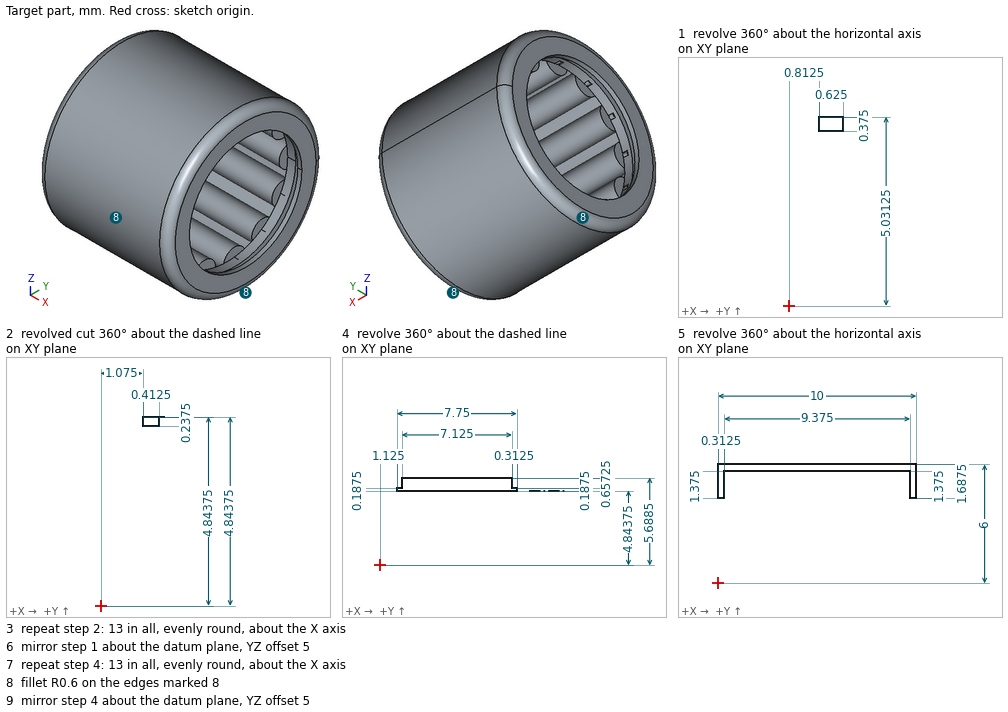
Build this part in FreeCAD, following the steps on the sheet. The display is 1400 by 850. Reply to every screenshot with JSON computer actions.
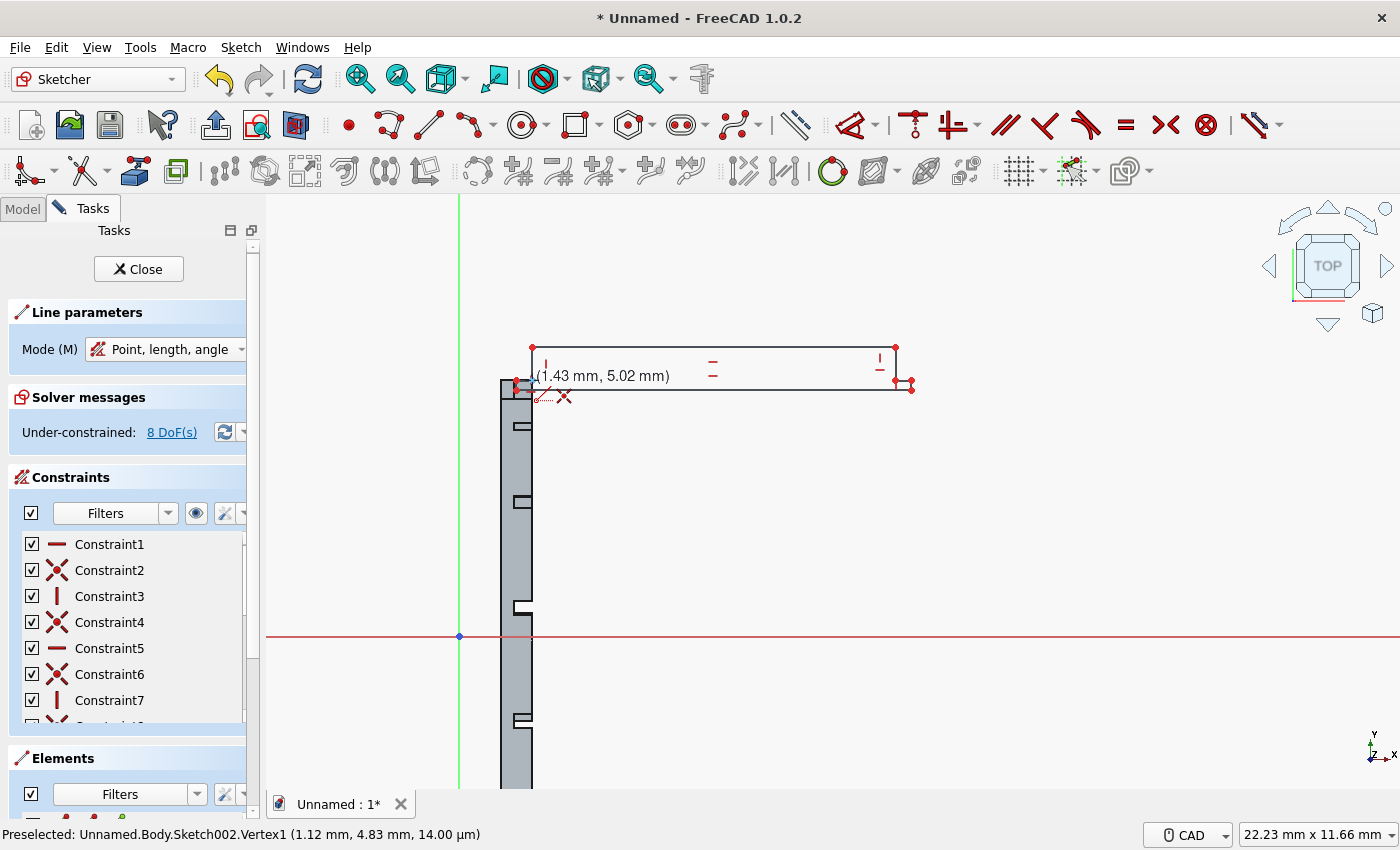
{"action": "left_click", "coordinate": [951, 390]}
{"action": "left_click", "coordinate": [1070, 390]}
{"action": "key", "text": "Escape"}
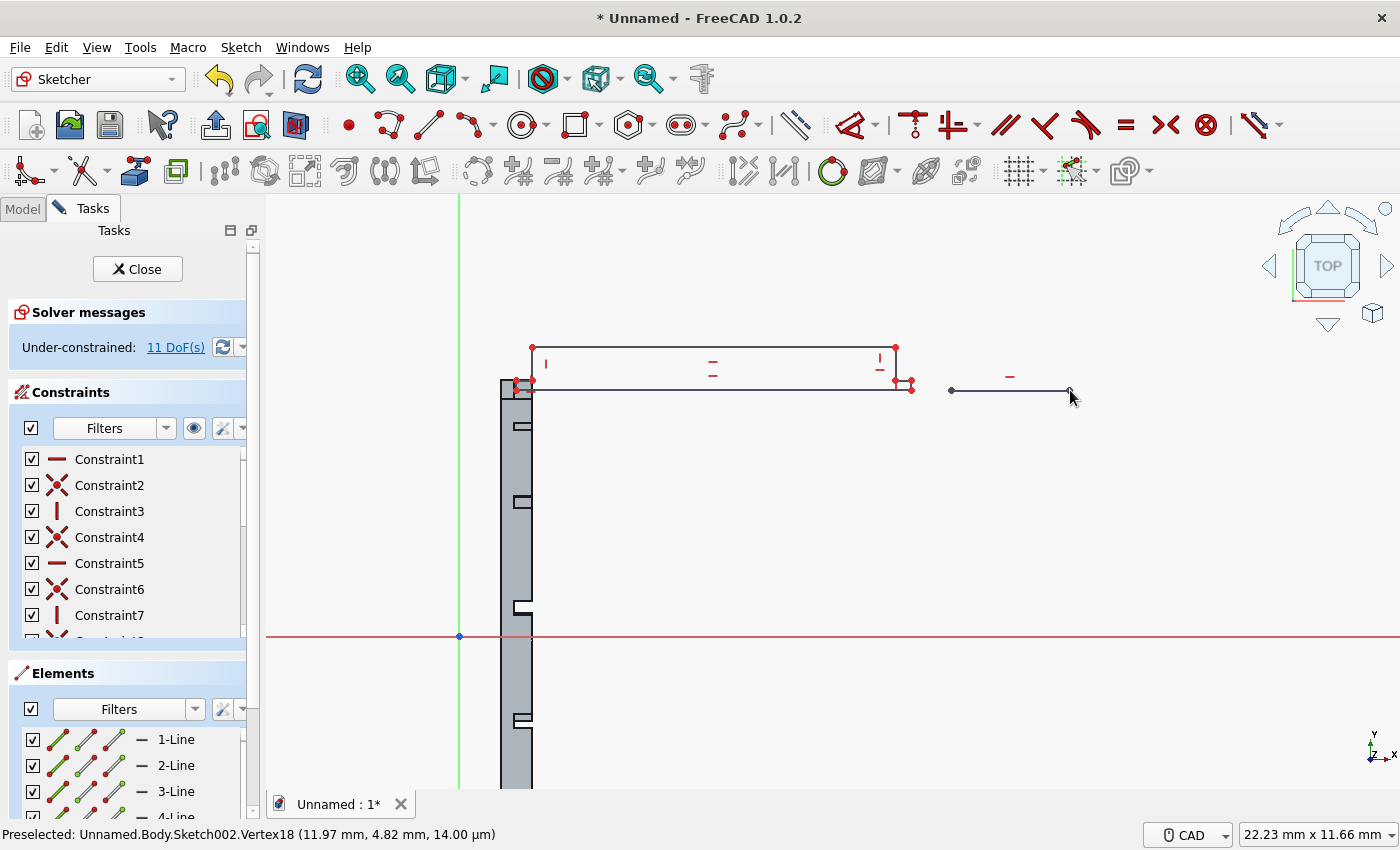
{"action": "left_click", "coordinate": [987, 391]}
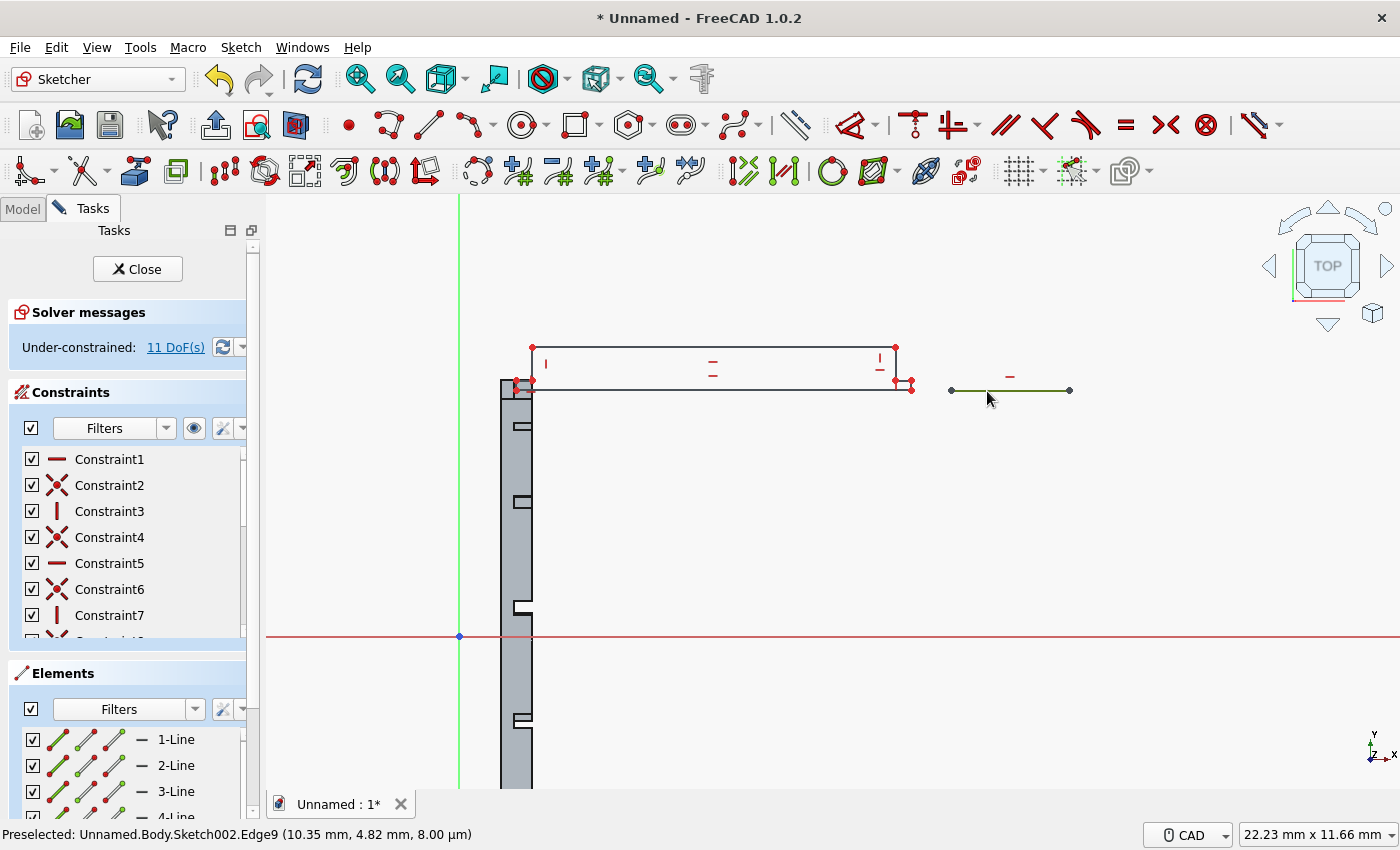
{"action": "key", "text": "g n"}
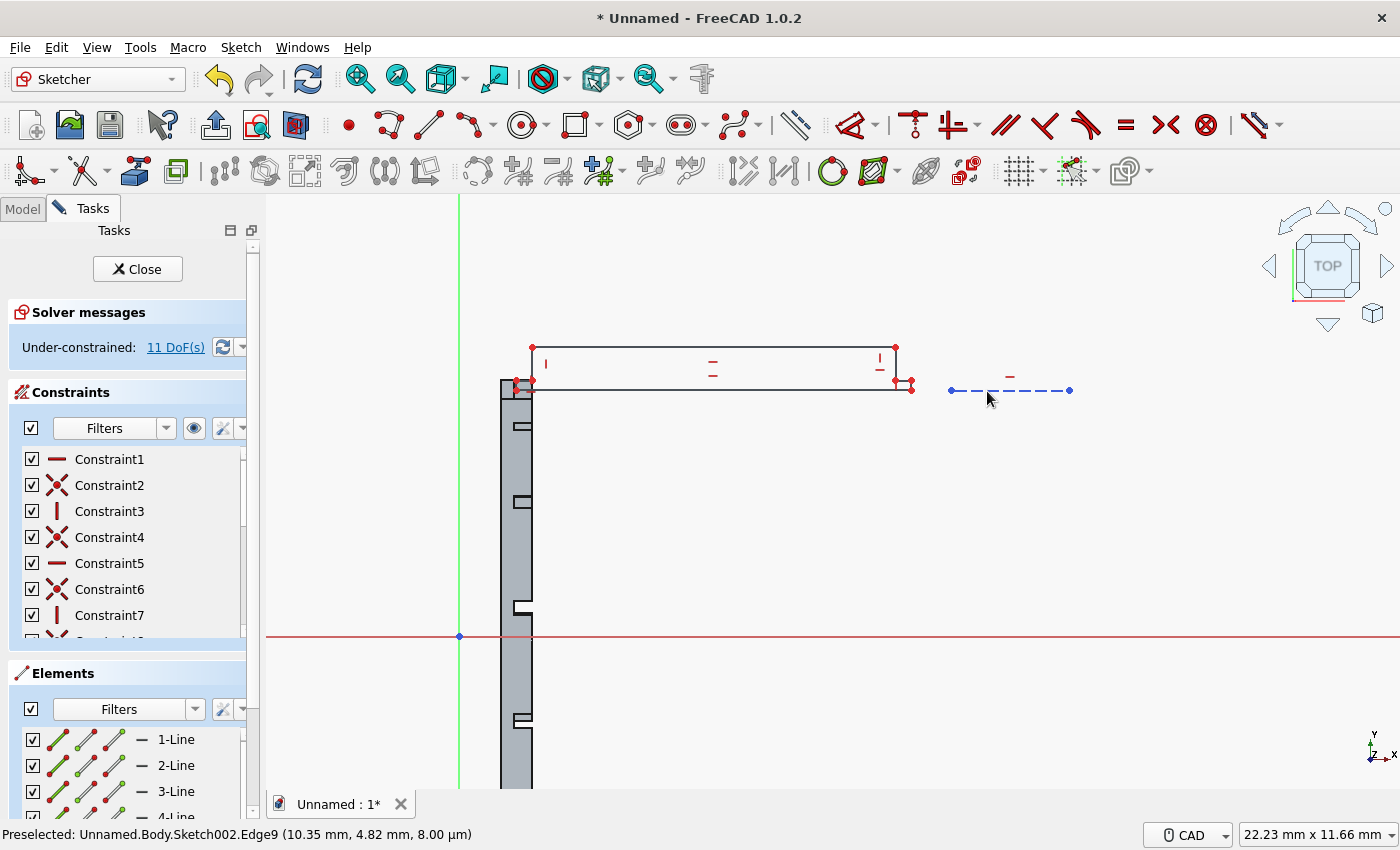
{"action": "key", "text": "d"}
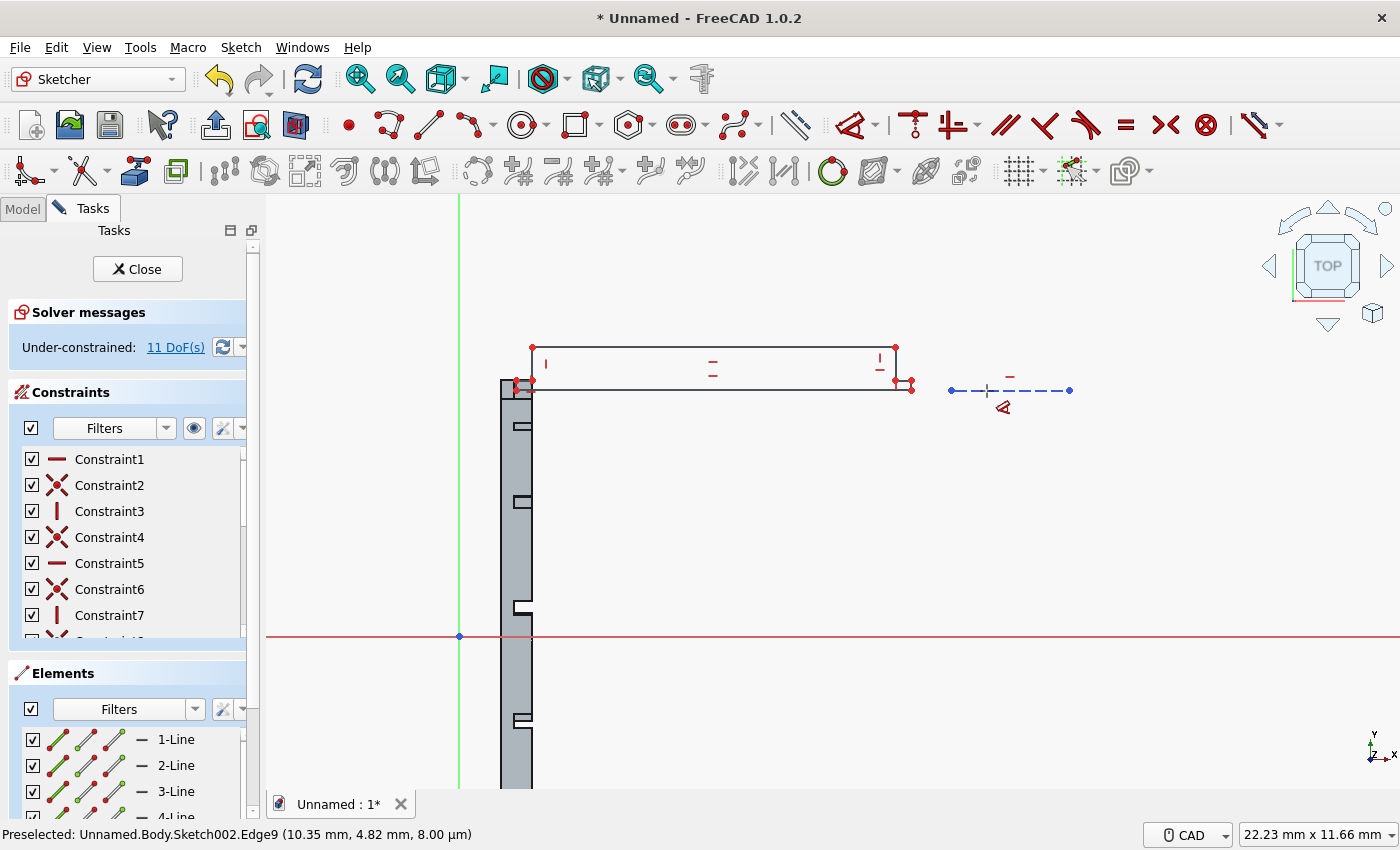
{"action": "left_click", "coordinate": [635, 390]}
{"action": "left_click", "coordinate": [714, 424]}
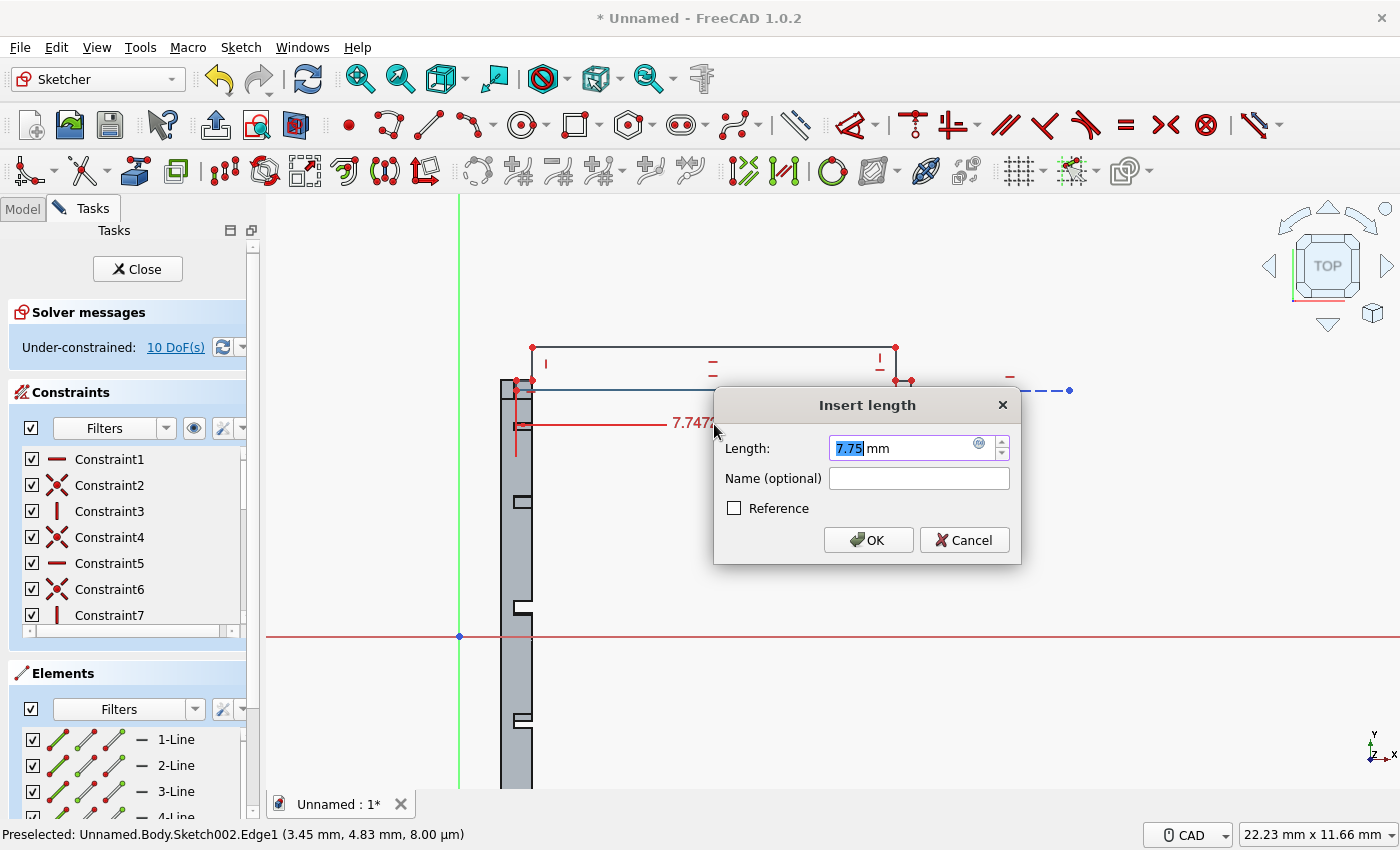
{"action": "type", "text": "7.75"}
{"action": "key", "text": "Return"}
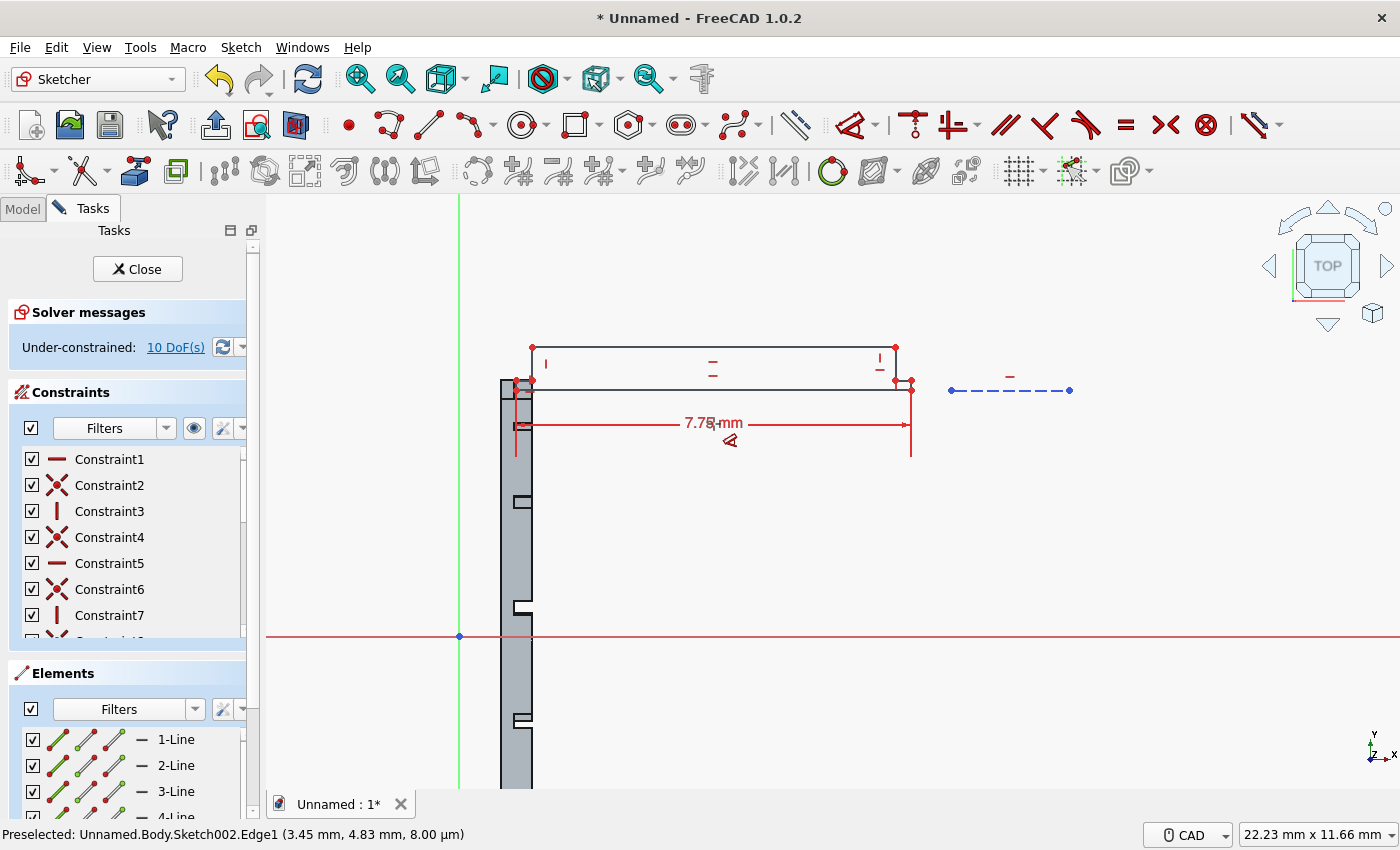
{"action": "left_click", "coordinate": [787, 347]}
{"action": "left_click", "coordinate": [714, 313]}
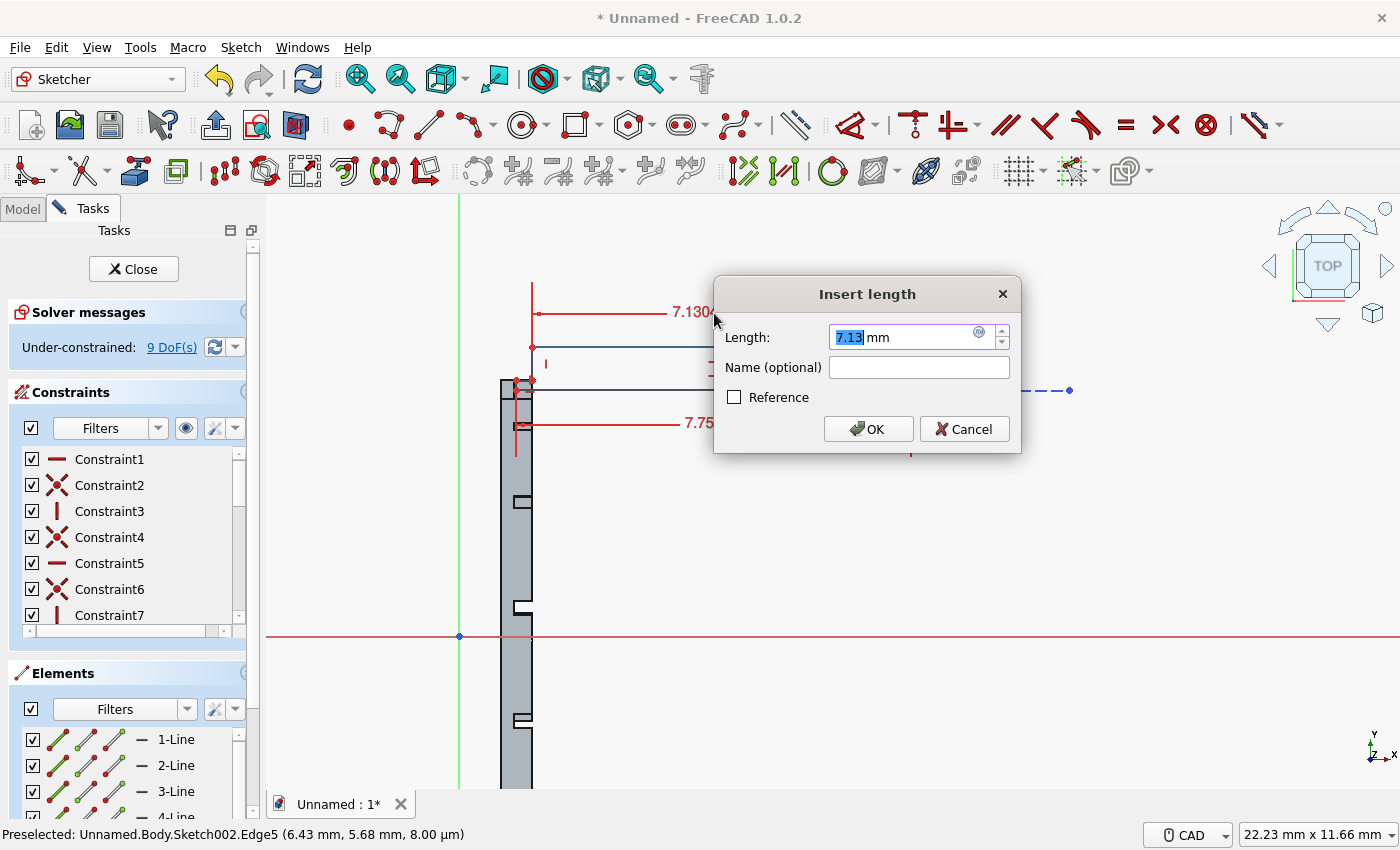
{"action": "type", "text": "7.125"}
{"action": "key", "text": "Return"}